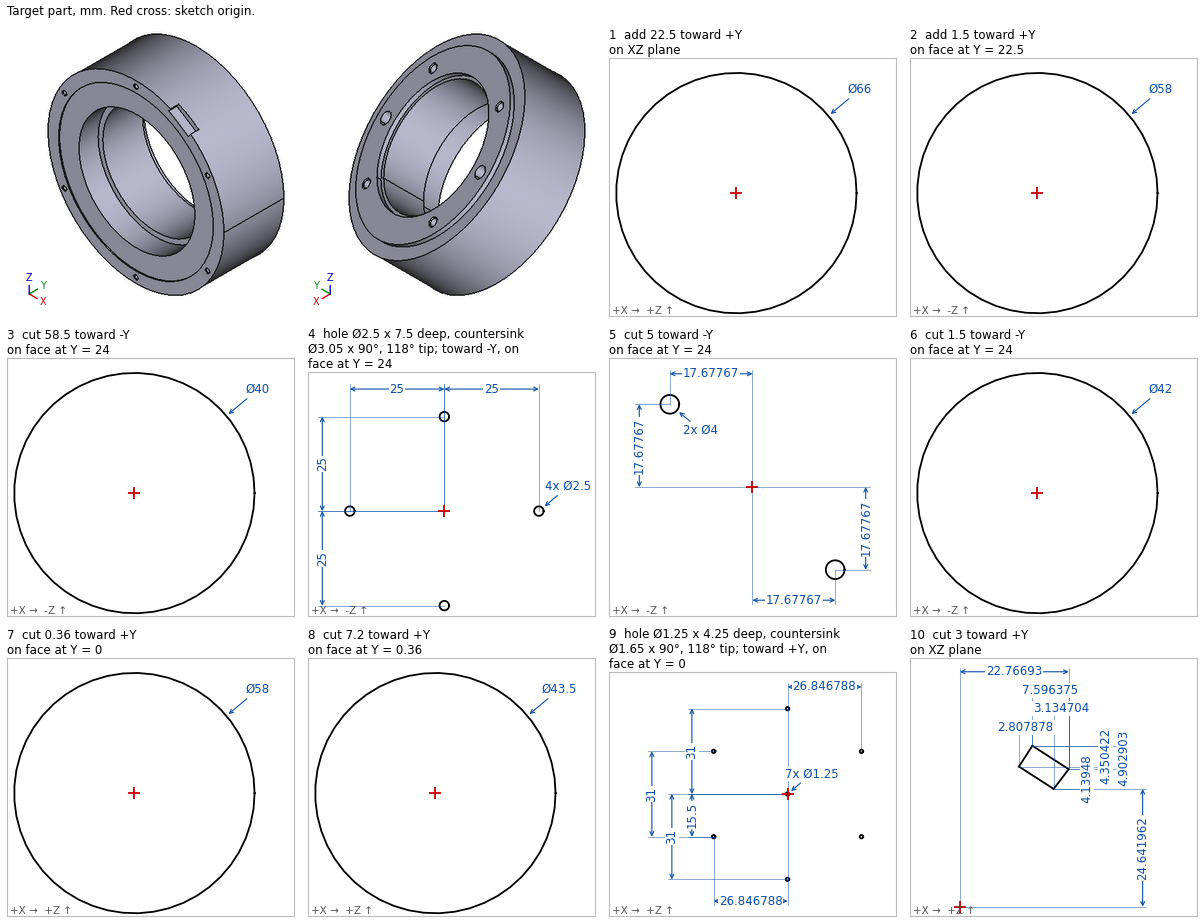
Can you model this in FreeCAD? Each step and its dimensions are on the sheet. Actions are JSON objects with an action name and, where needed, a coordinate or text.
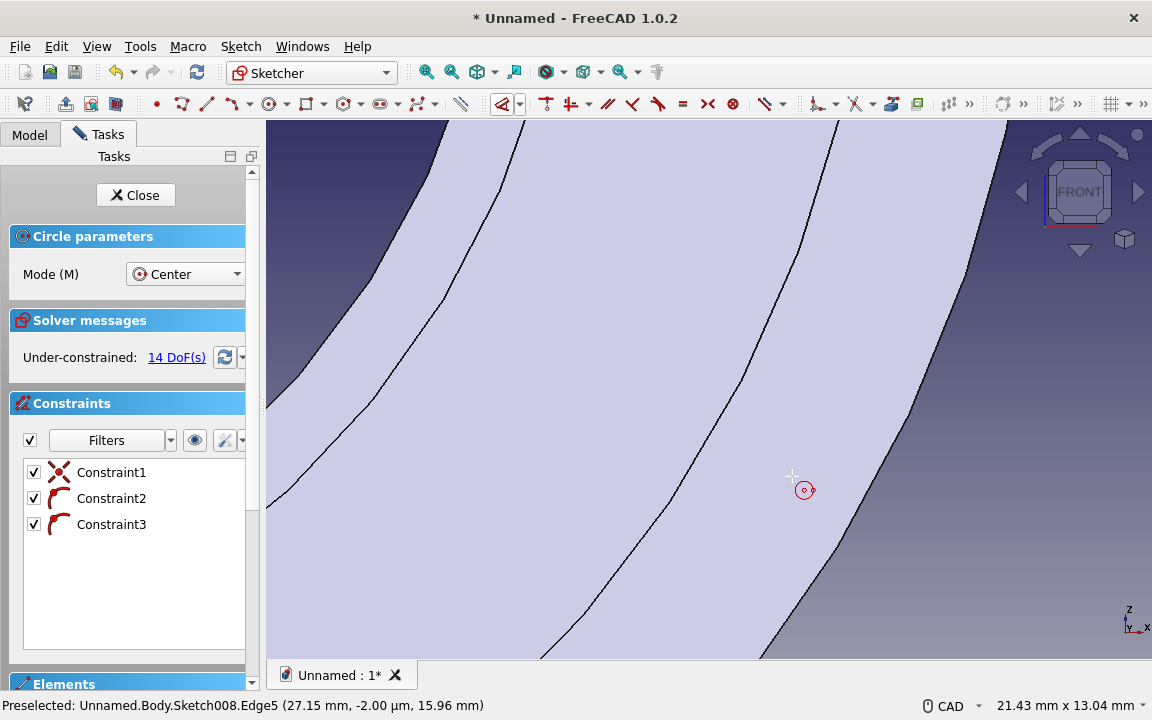
{"action": "scroll", "coordinate": [792, 477], "scroll_direction": "down", "scroll_amount": 10}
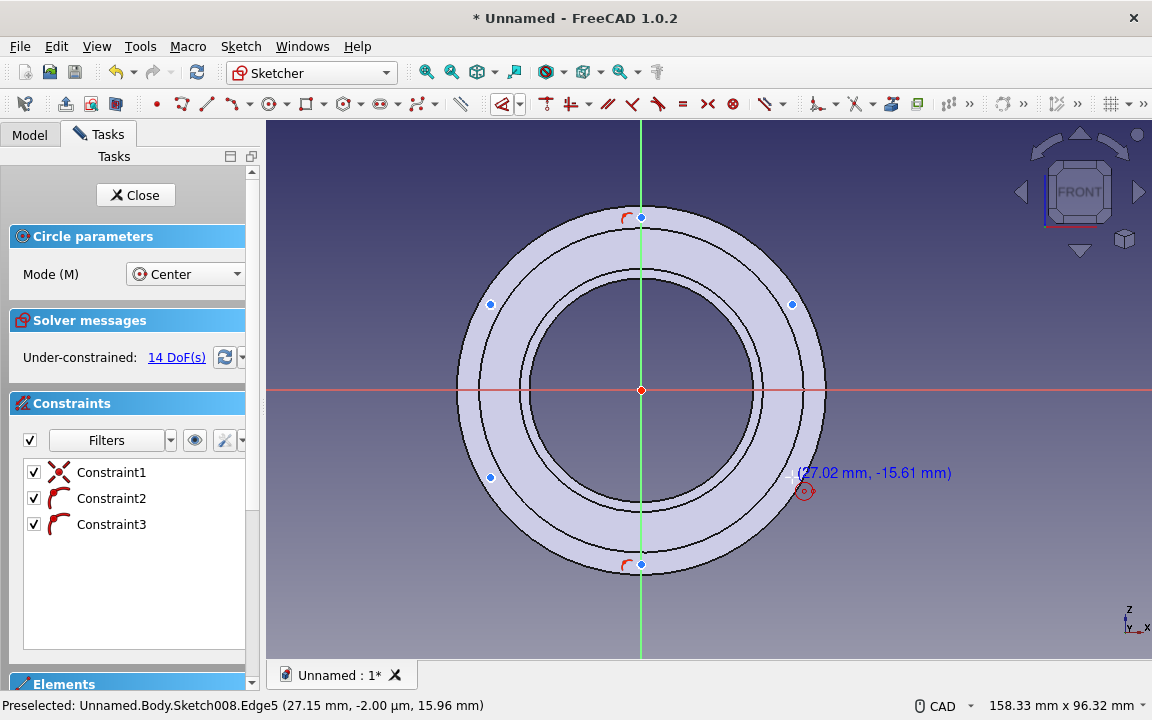
{"action": "left_click", "coordinate": [792, 477]}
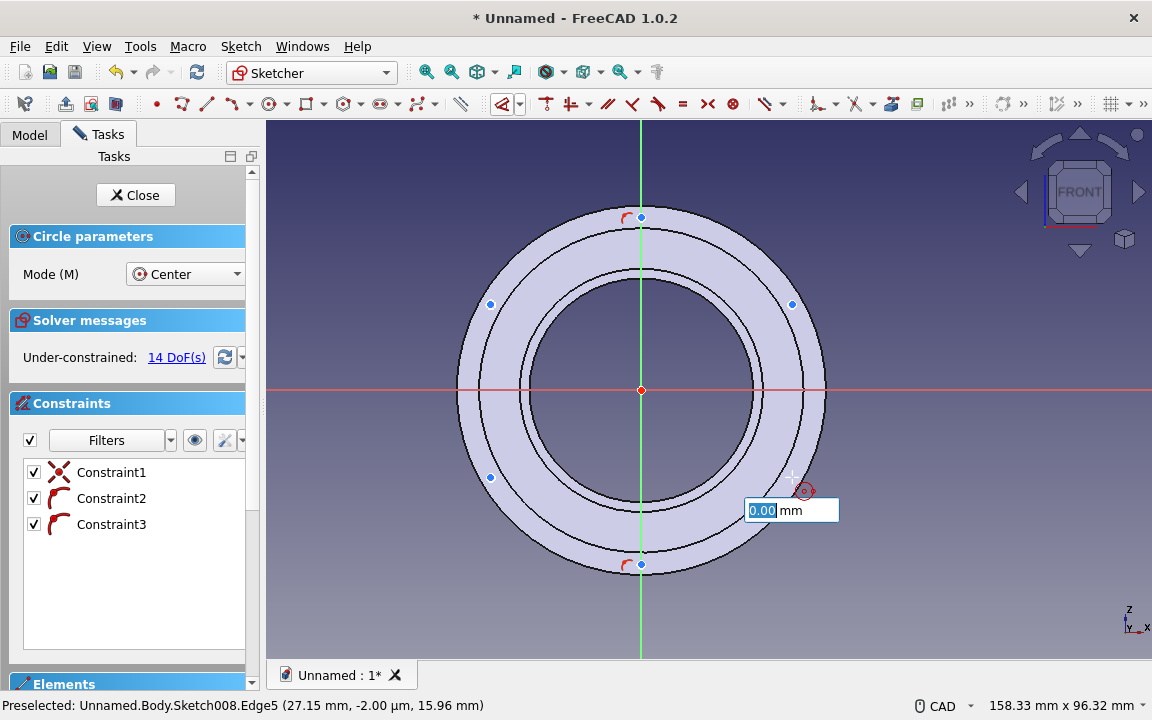
{"action": "scroll", "coordinate": [794, 475], "scroll_direction": "up", "scroll_amount": 8}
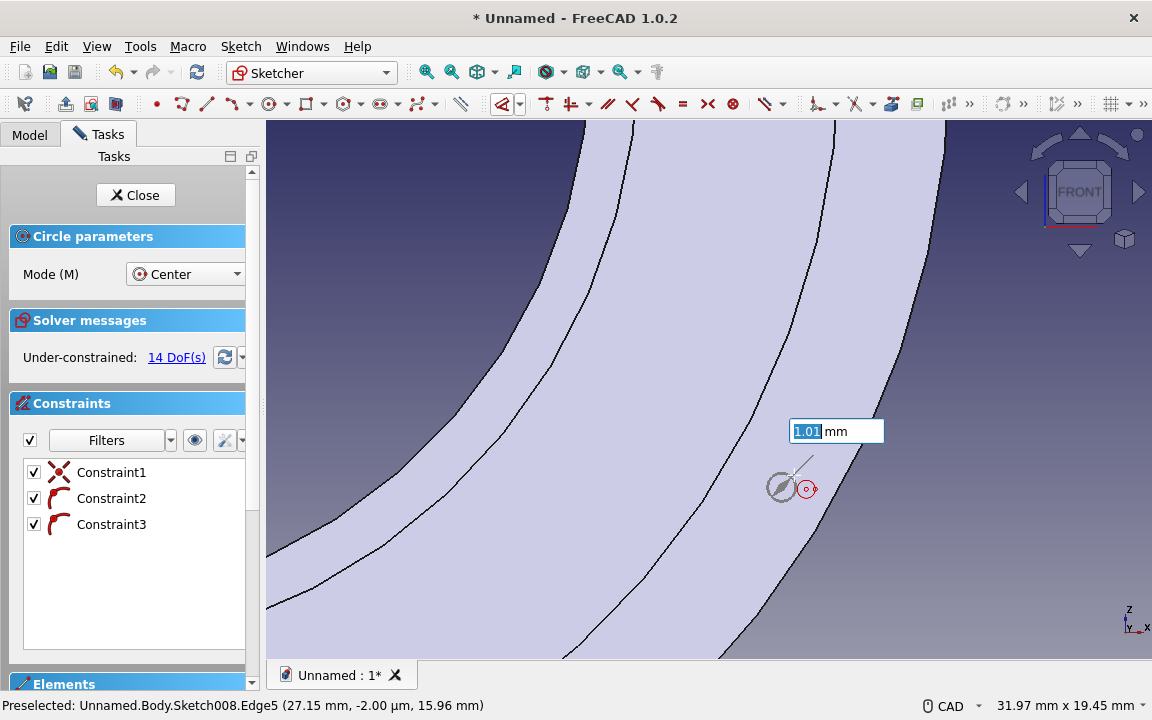
{"action": "left_click", "coordinate": [792, 471]}
{"action": "key", "text": "Escape"}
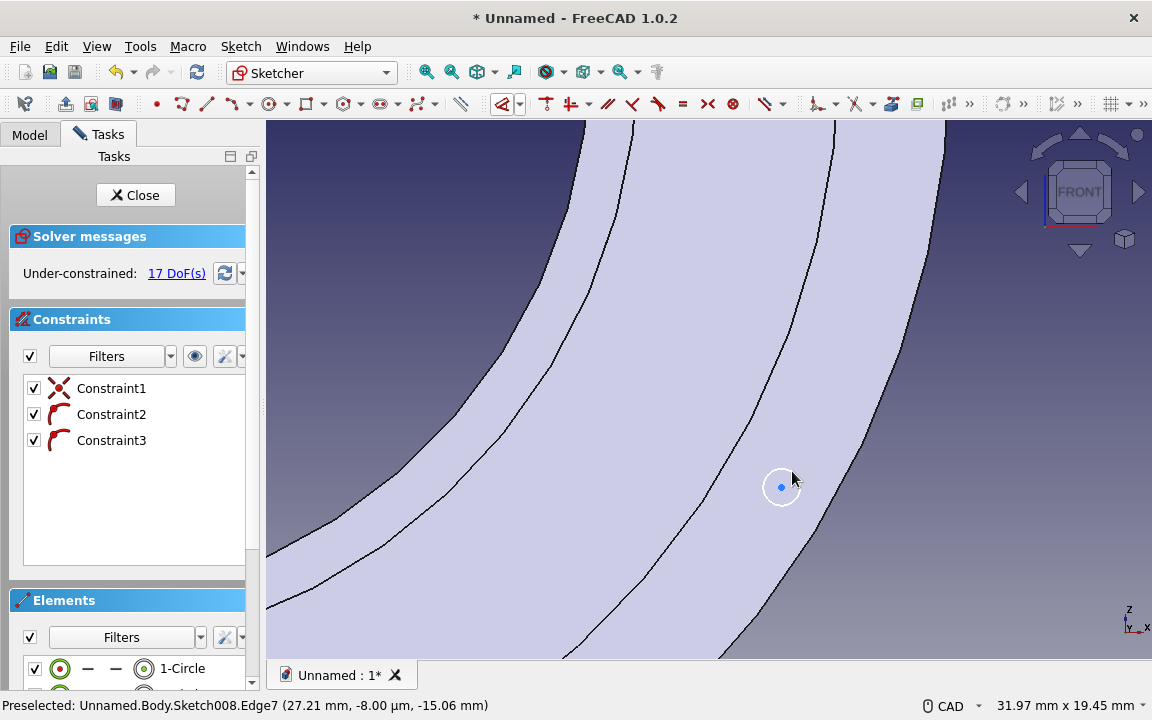
{"action": "scroll", "coordinate": [794, 475], "scroll_direction": "down", "scroll_amount": 8}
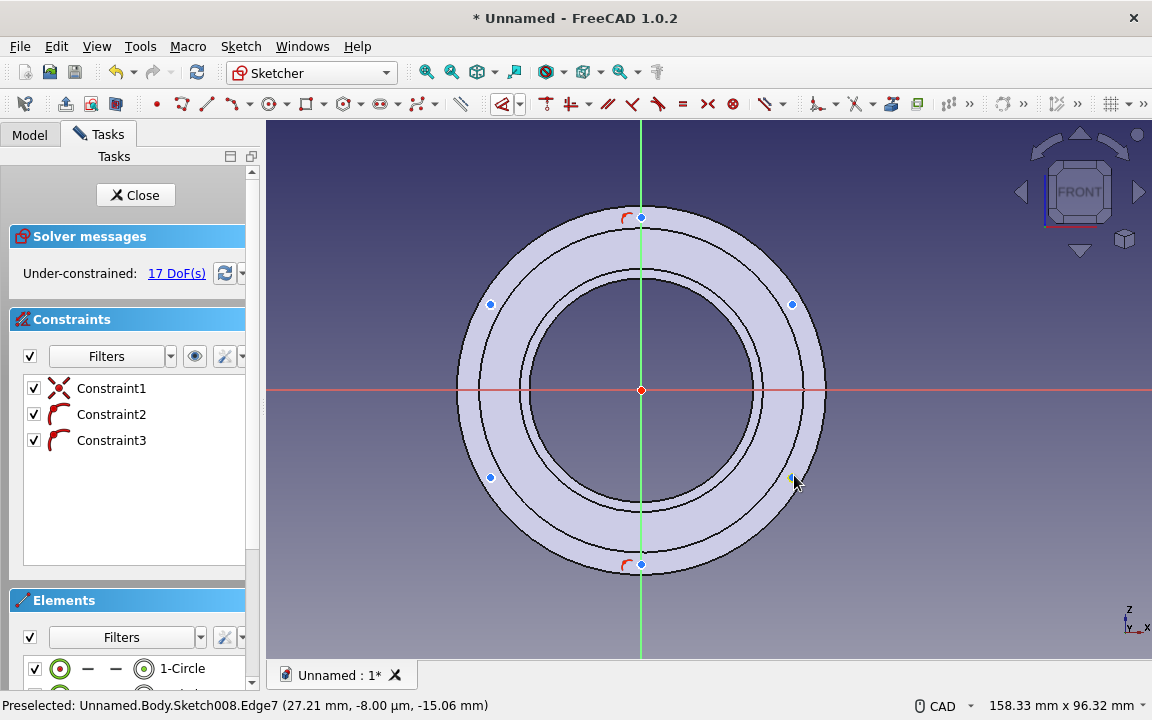
{"action": "scroll", "coordinate": [644, 388], "scroll_direction": "up", "scroll_amount": 9}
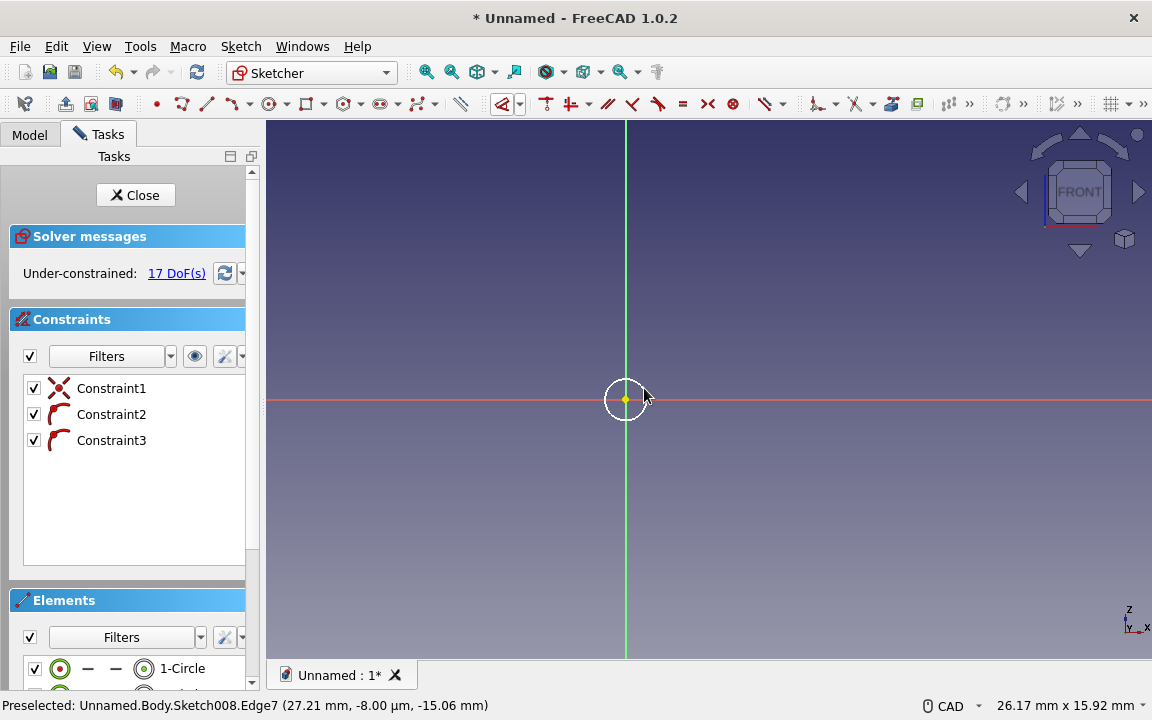
{"action": "left_click", "coordinate": [640, 385]}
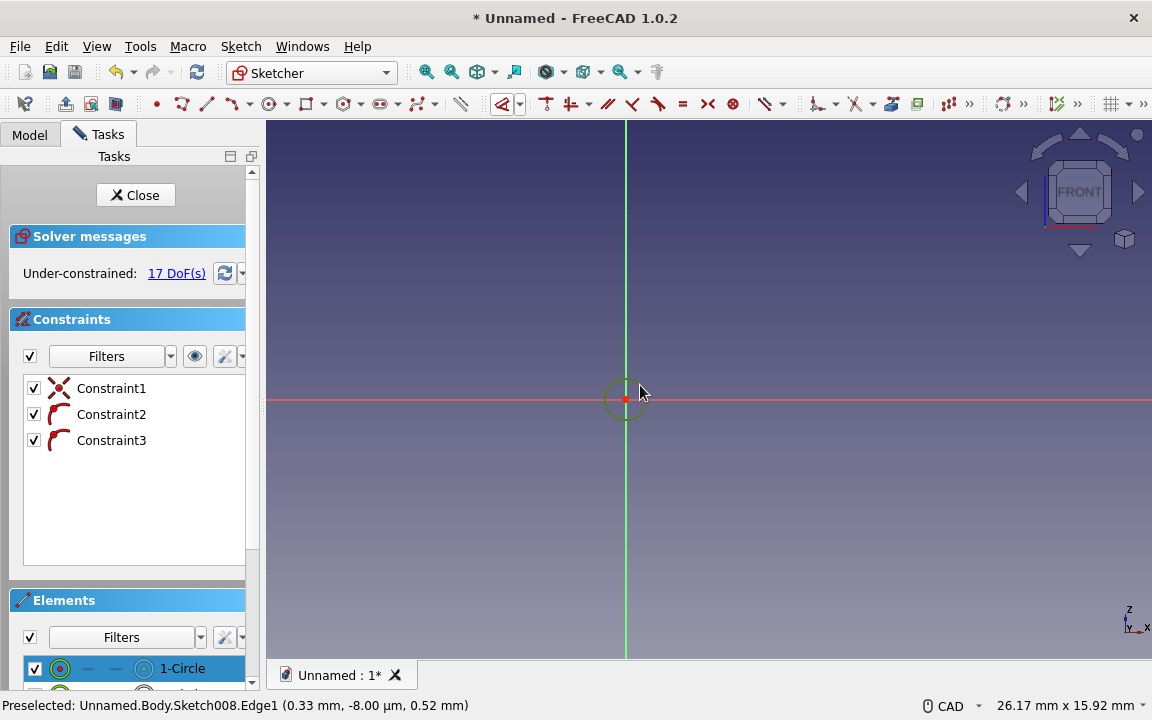
{"action": "scroll", "coordinate": [643, 387], "scroll_direction": "down", "scroll_amount": 9}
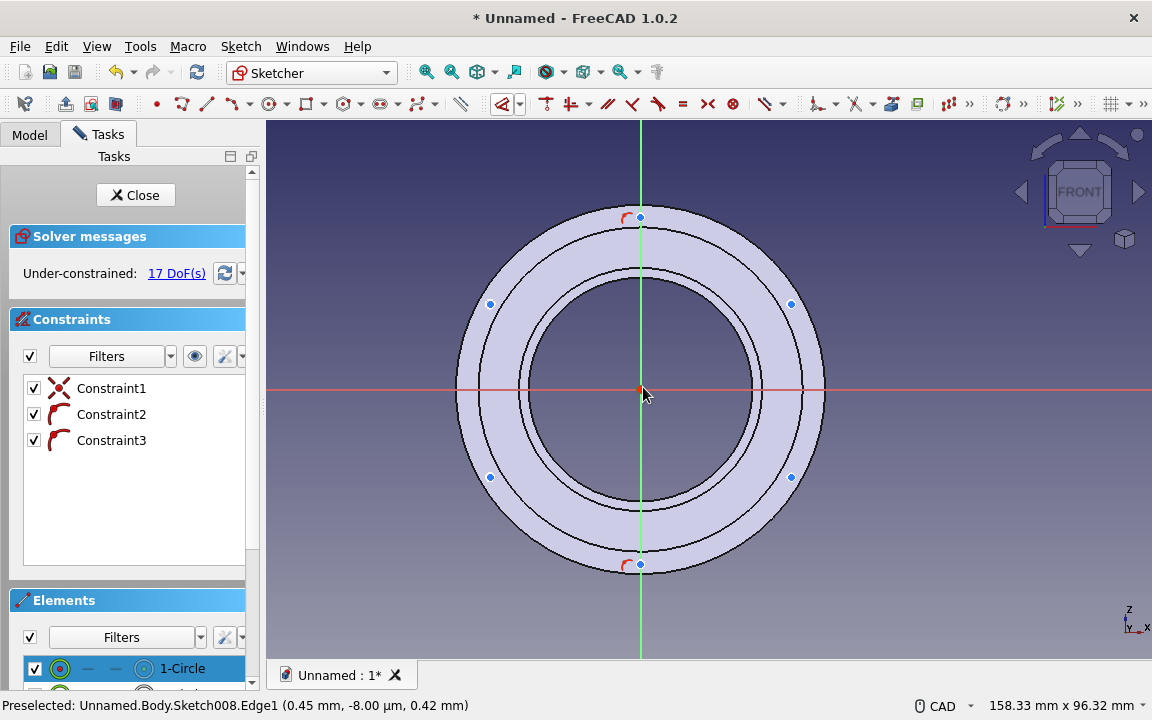
{"action": "scroll", "coordinate": [643, 561], "scroll_direction": "up", "scroll_amount": 9}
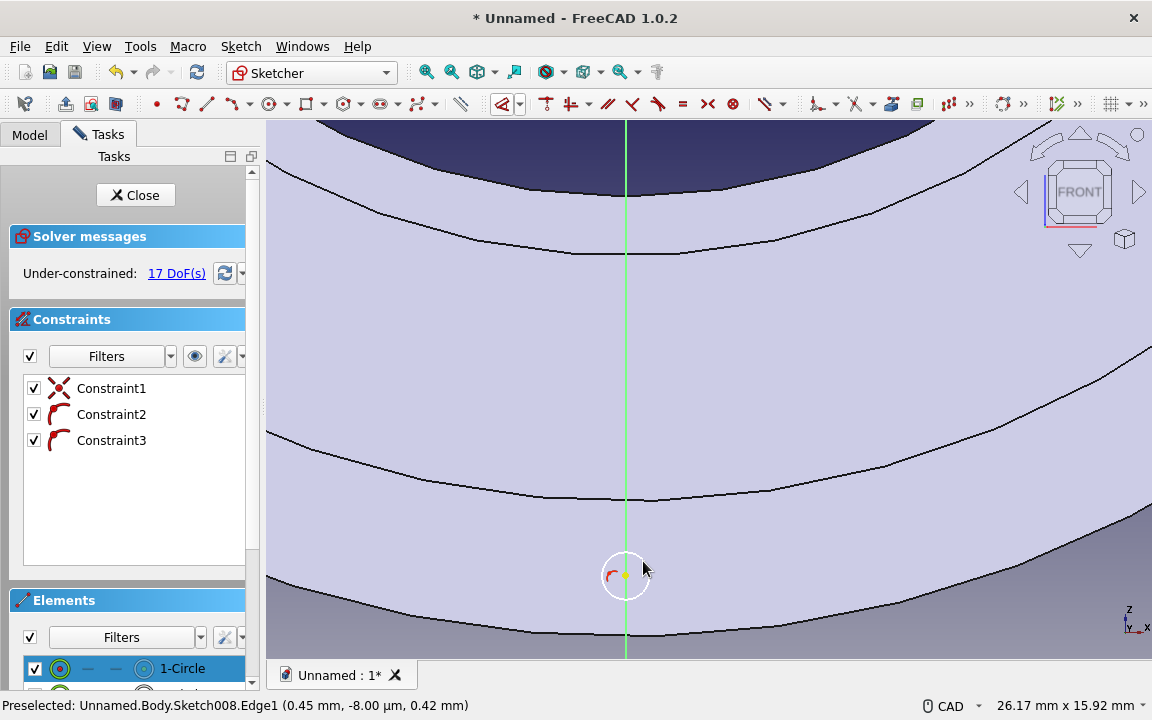
{"action": "left_click", "coordinate": [642, 559]}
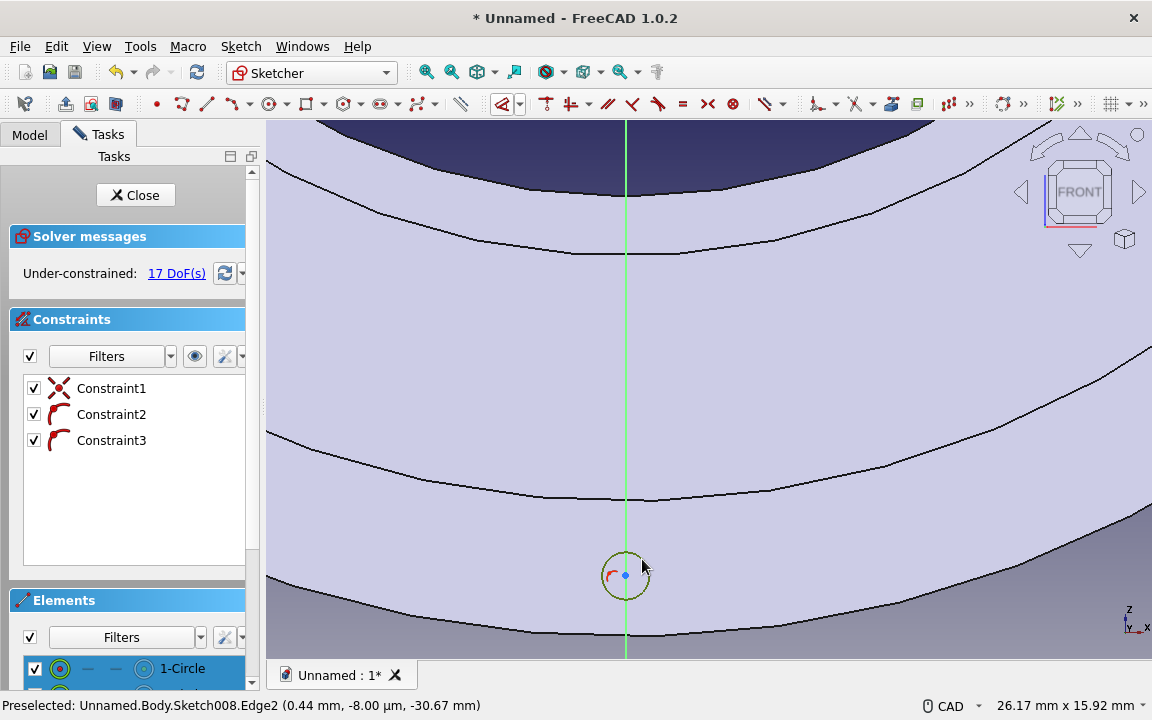
{"action": "scroll", "coordinate": [643, 562], "scroll_direction": "down", "scroll_amount": 9}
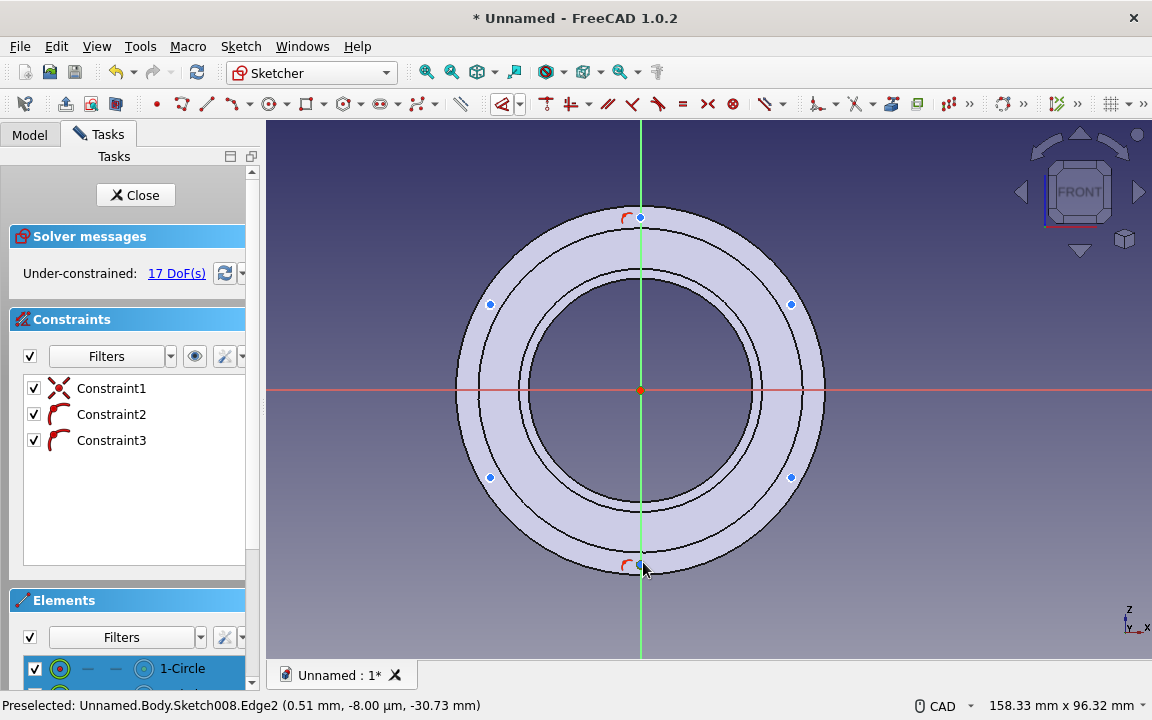
{"action": "scroll", "coordinate": [493, 475], "scroll_direction": "up", "scroll_amount": 6}